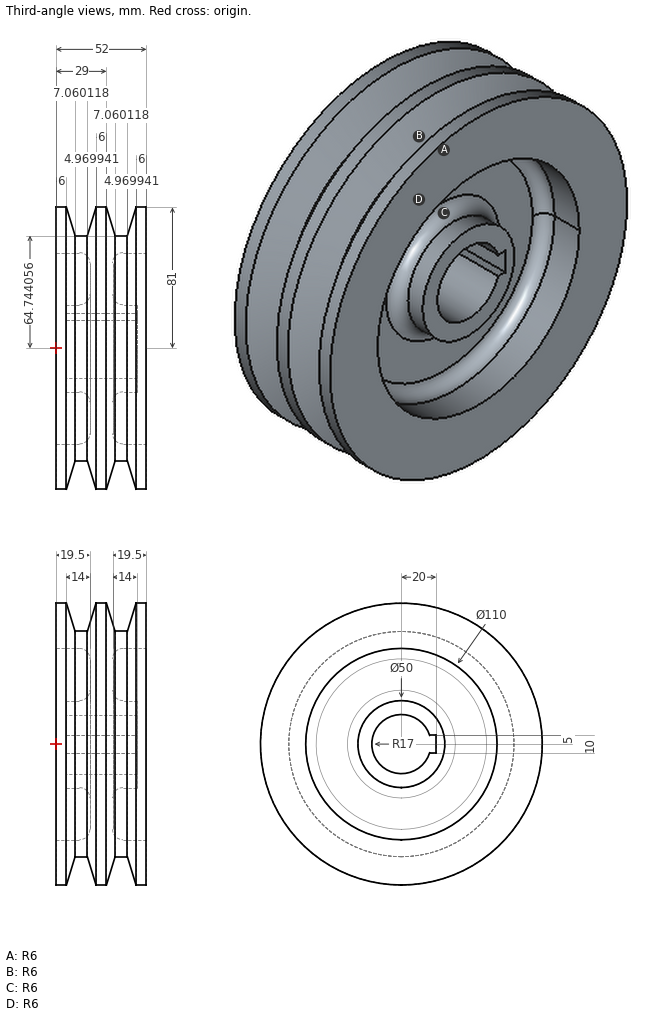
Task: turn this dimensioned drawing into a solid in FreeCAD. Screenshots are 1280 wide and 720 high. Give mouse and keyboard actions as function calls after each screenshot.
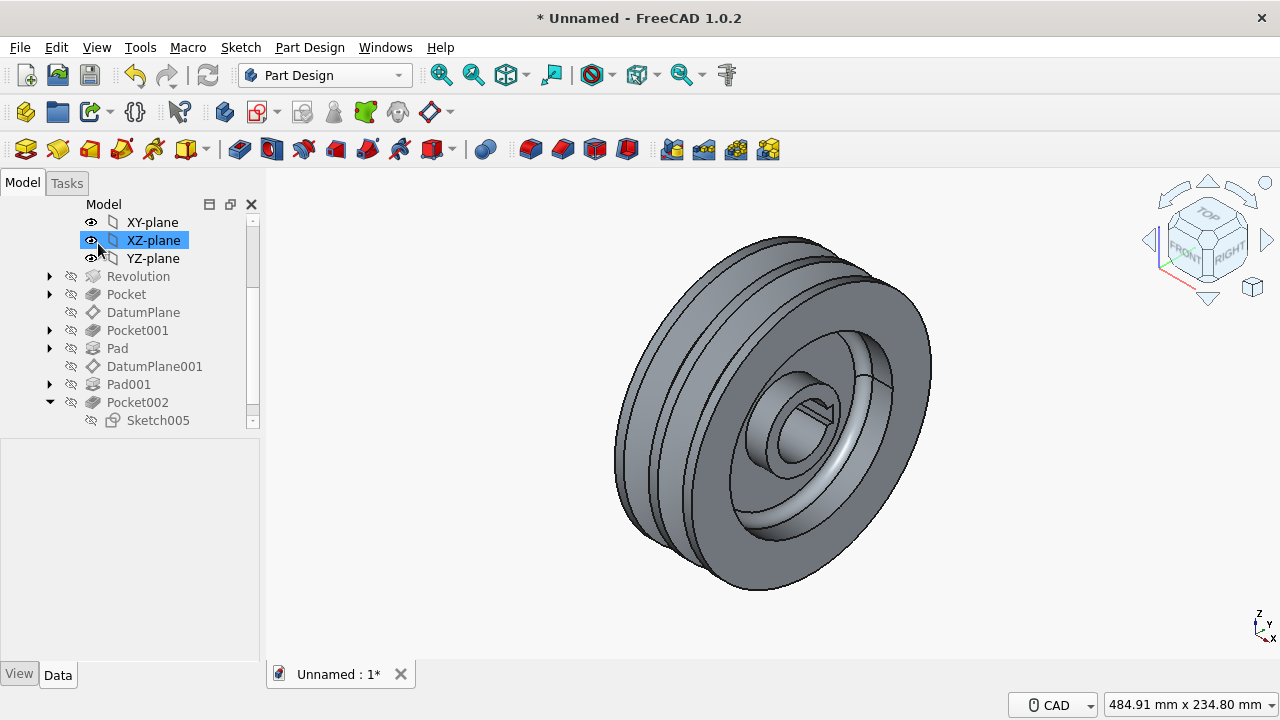
key(2)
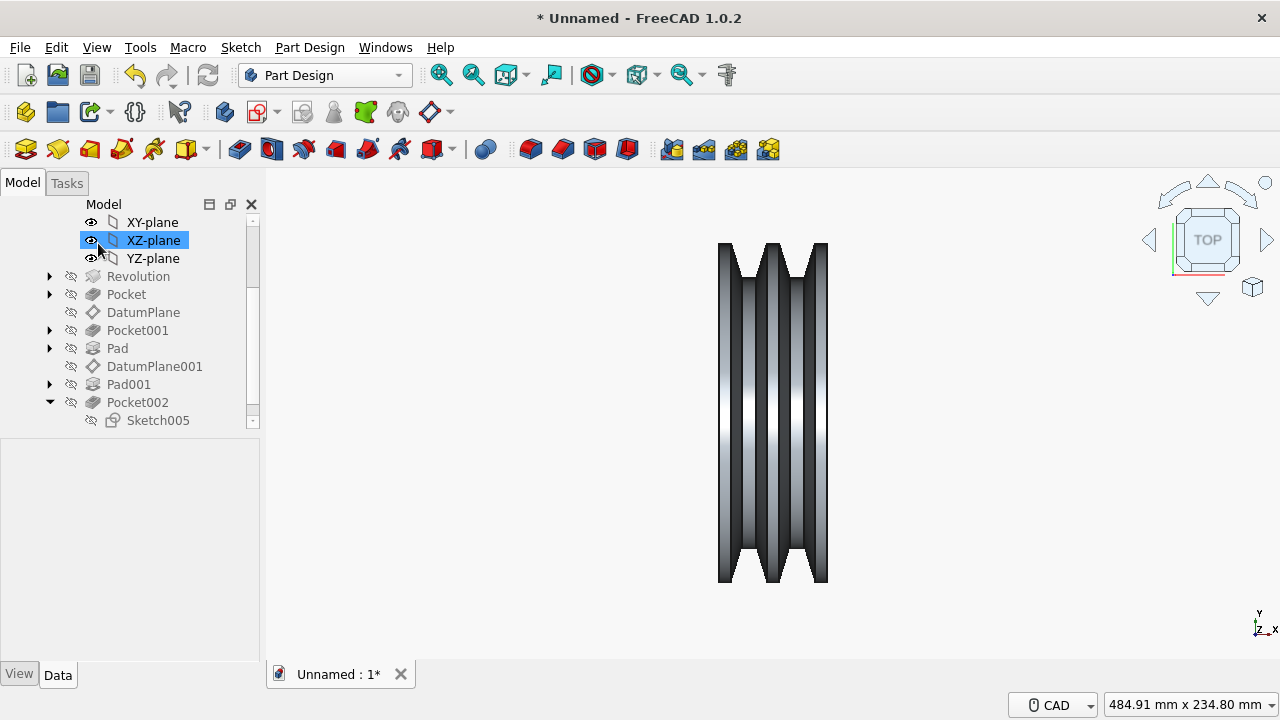
key(0)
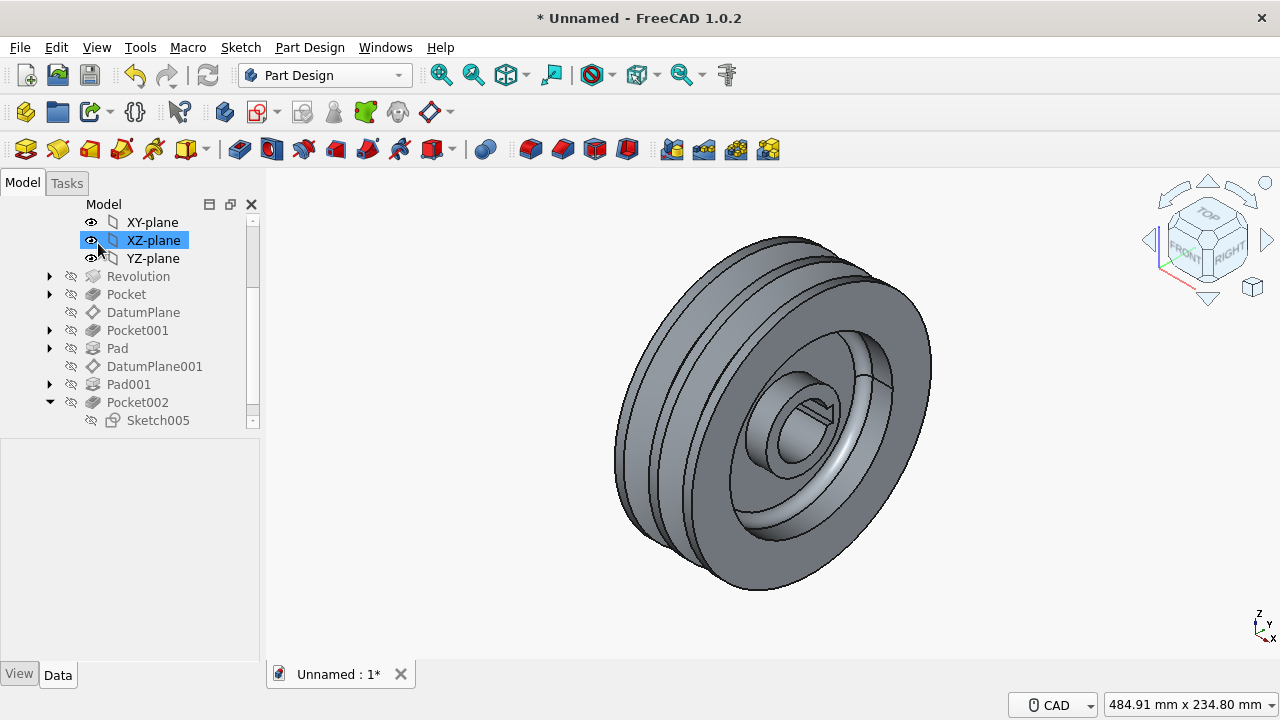
key(1)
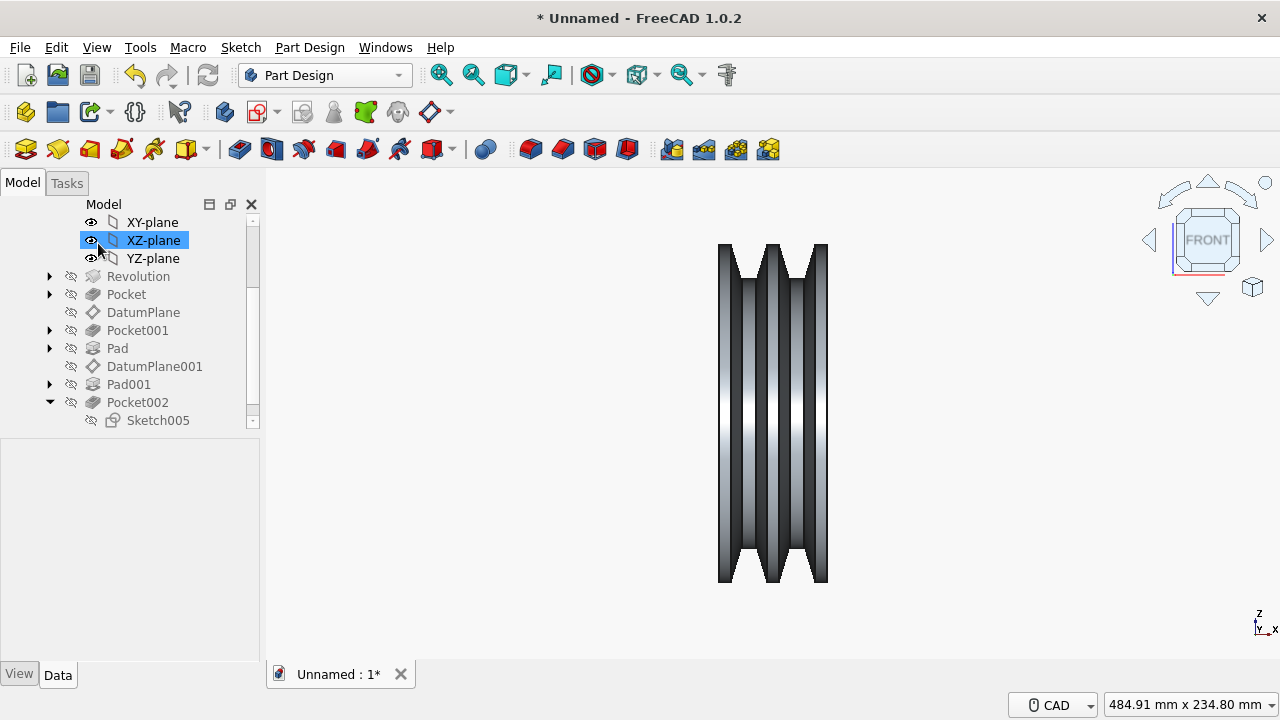
key(3)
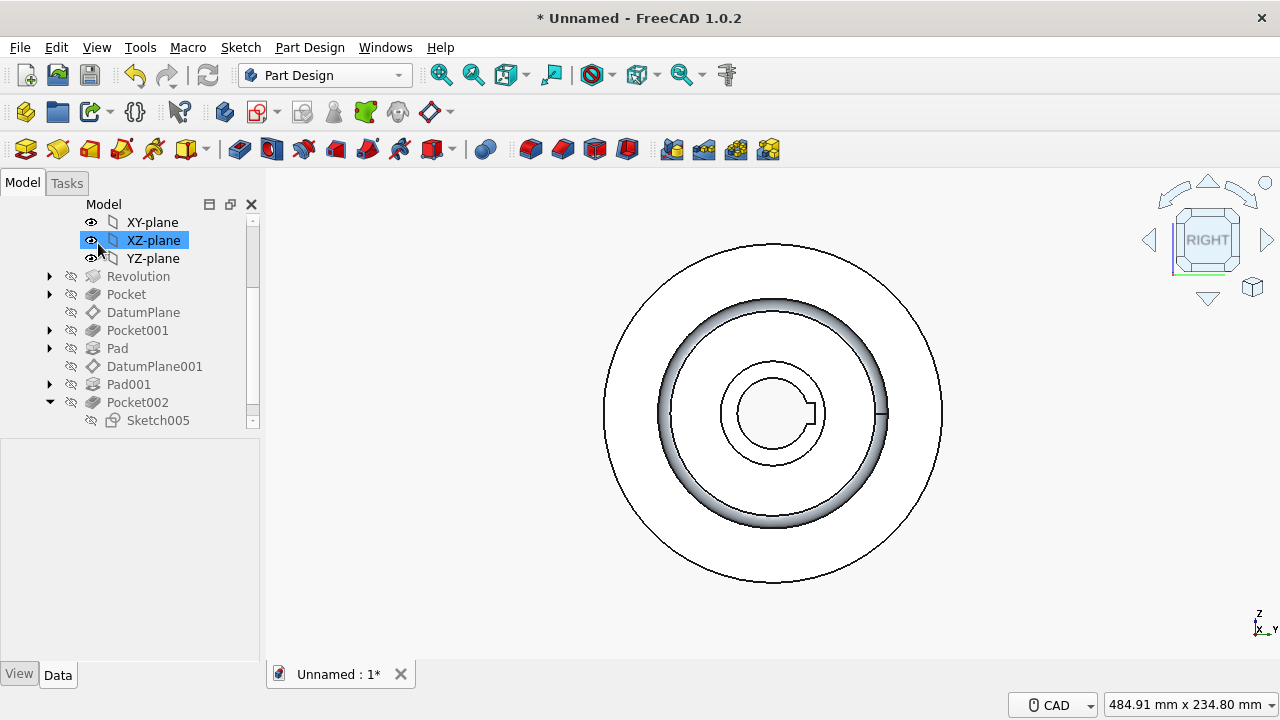
key(5)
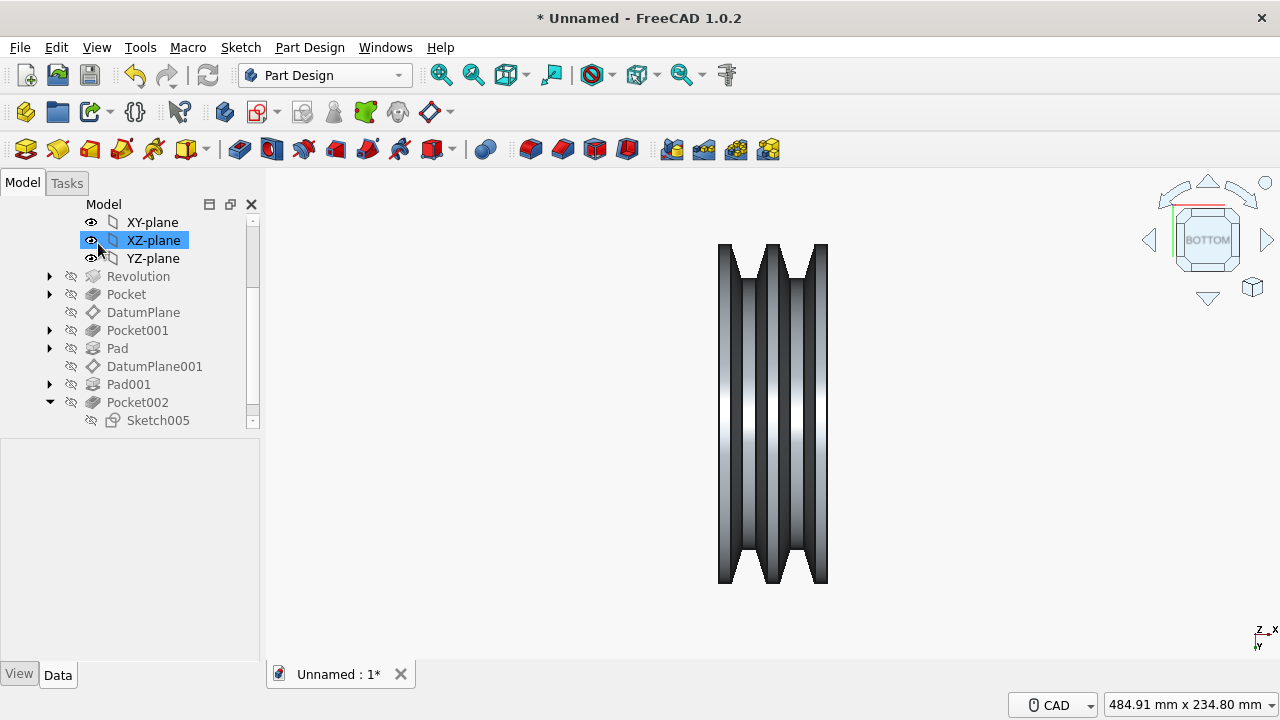
key(4)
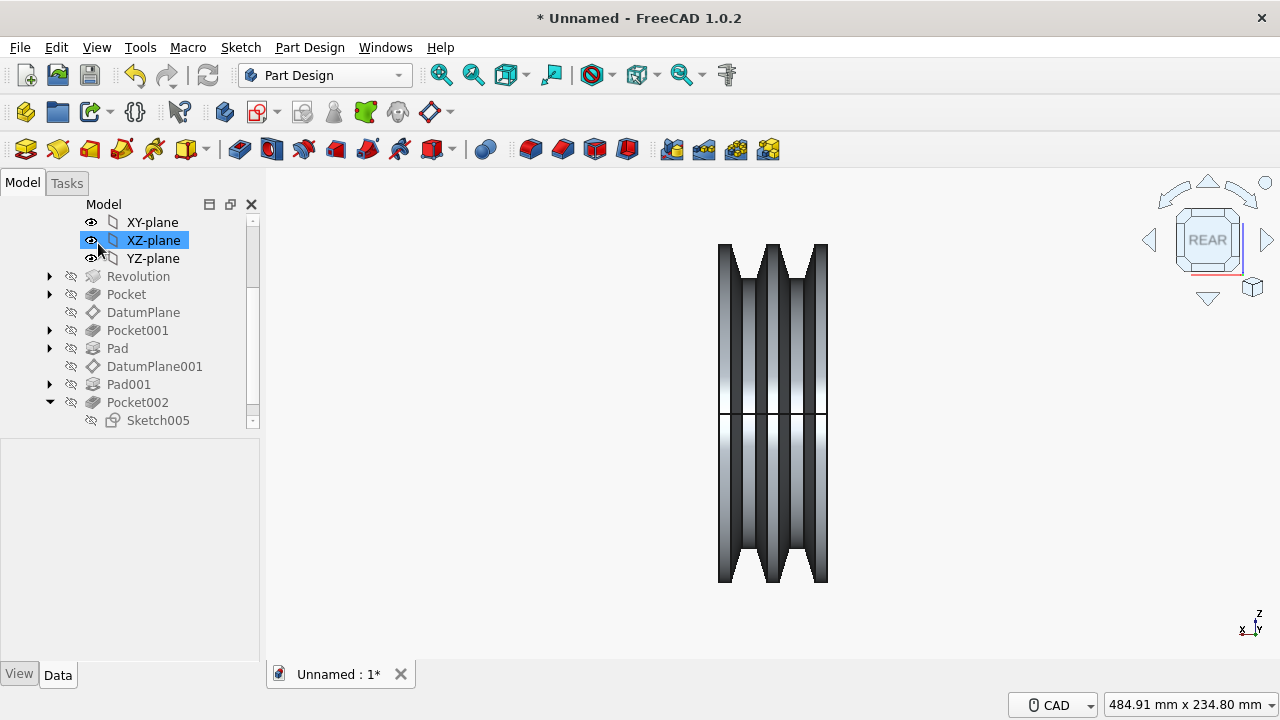
key(6)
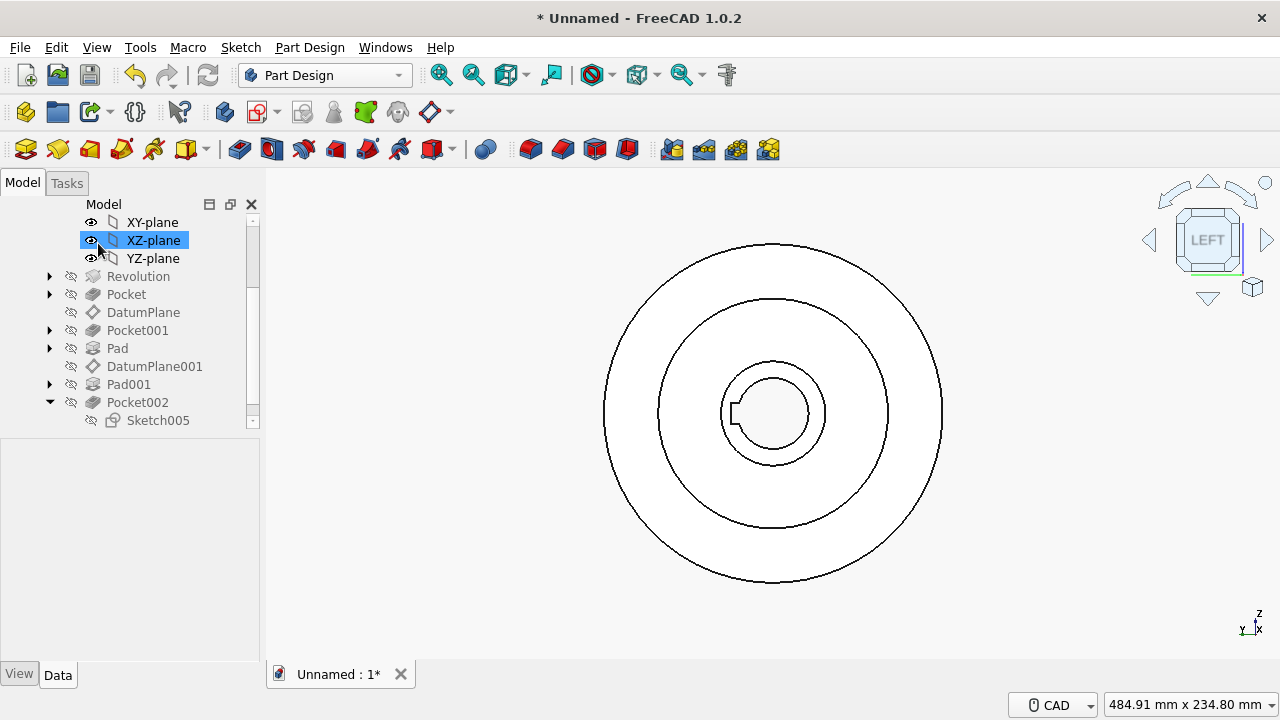
key(v)
key(3)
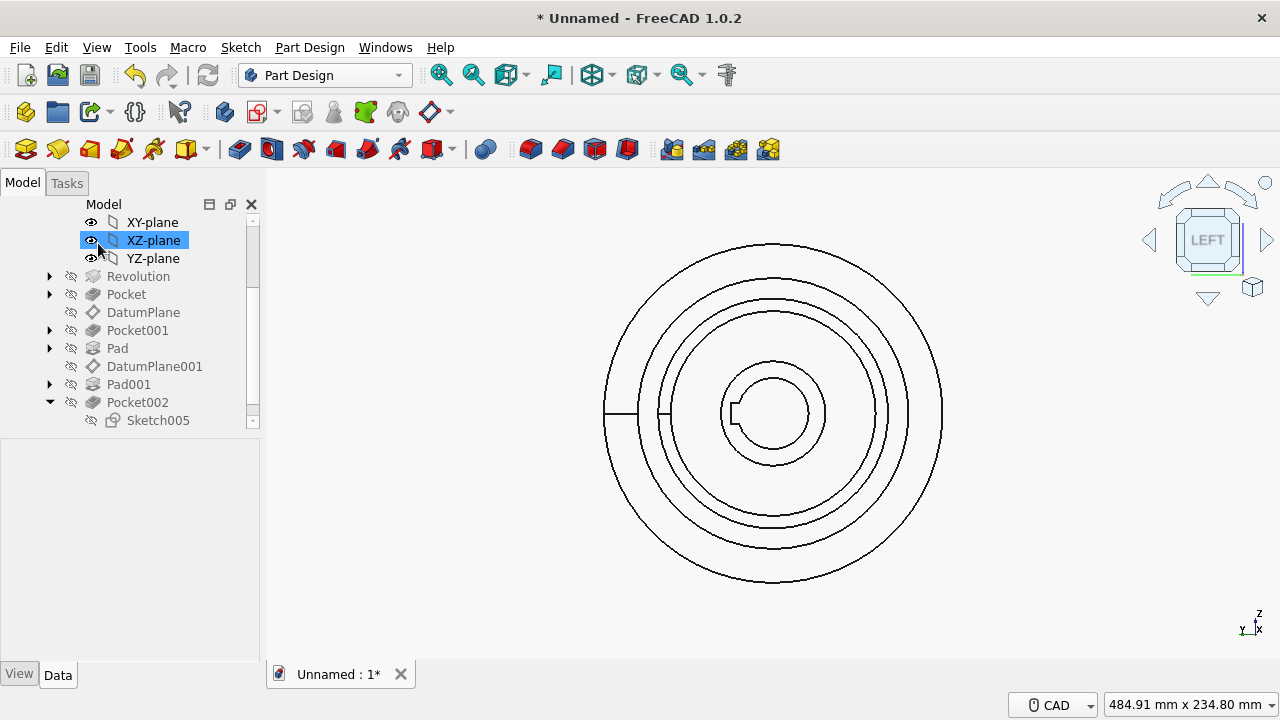
key(0)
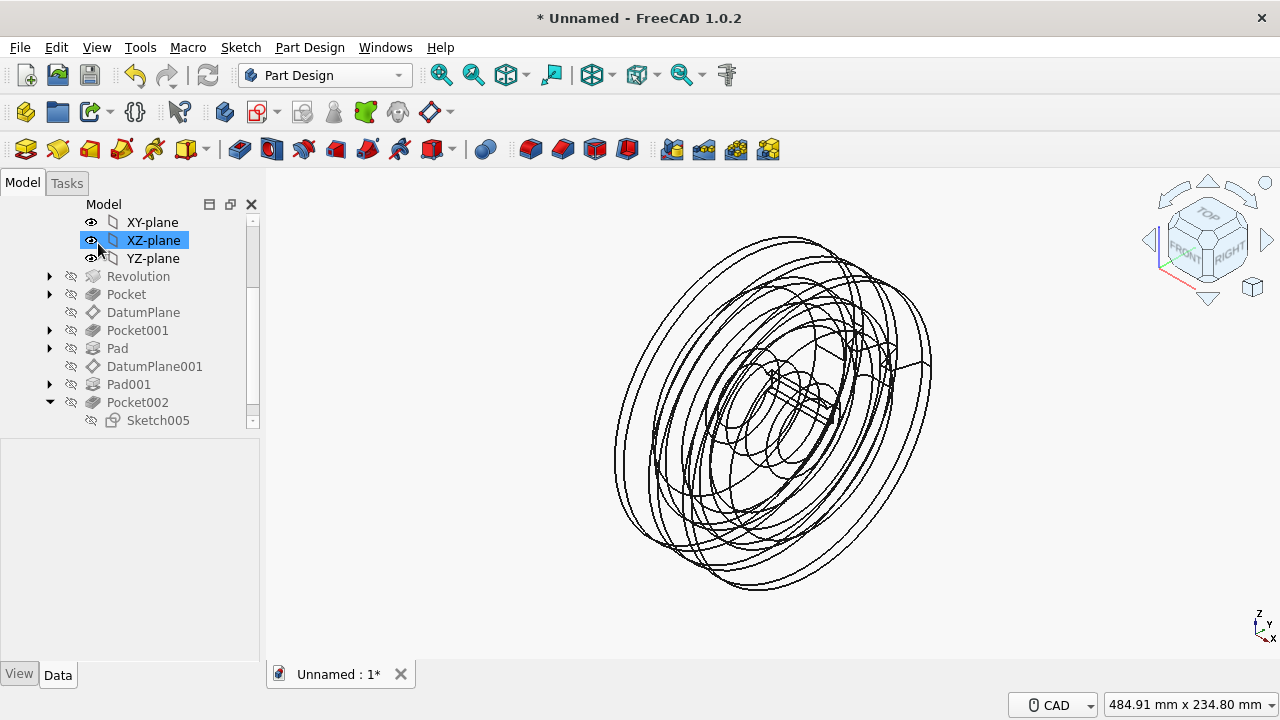
click(698, 390)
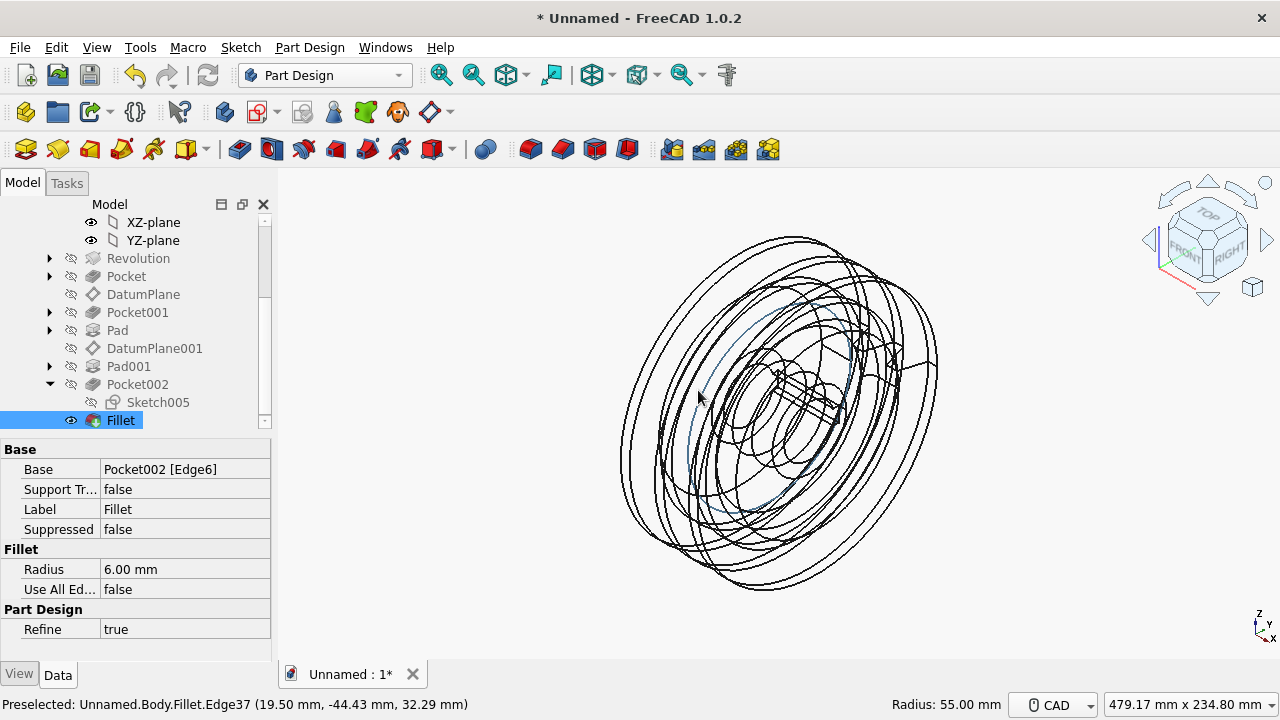
key(v)
key(1)